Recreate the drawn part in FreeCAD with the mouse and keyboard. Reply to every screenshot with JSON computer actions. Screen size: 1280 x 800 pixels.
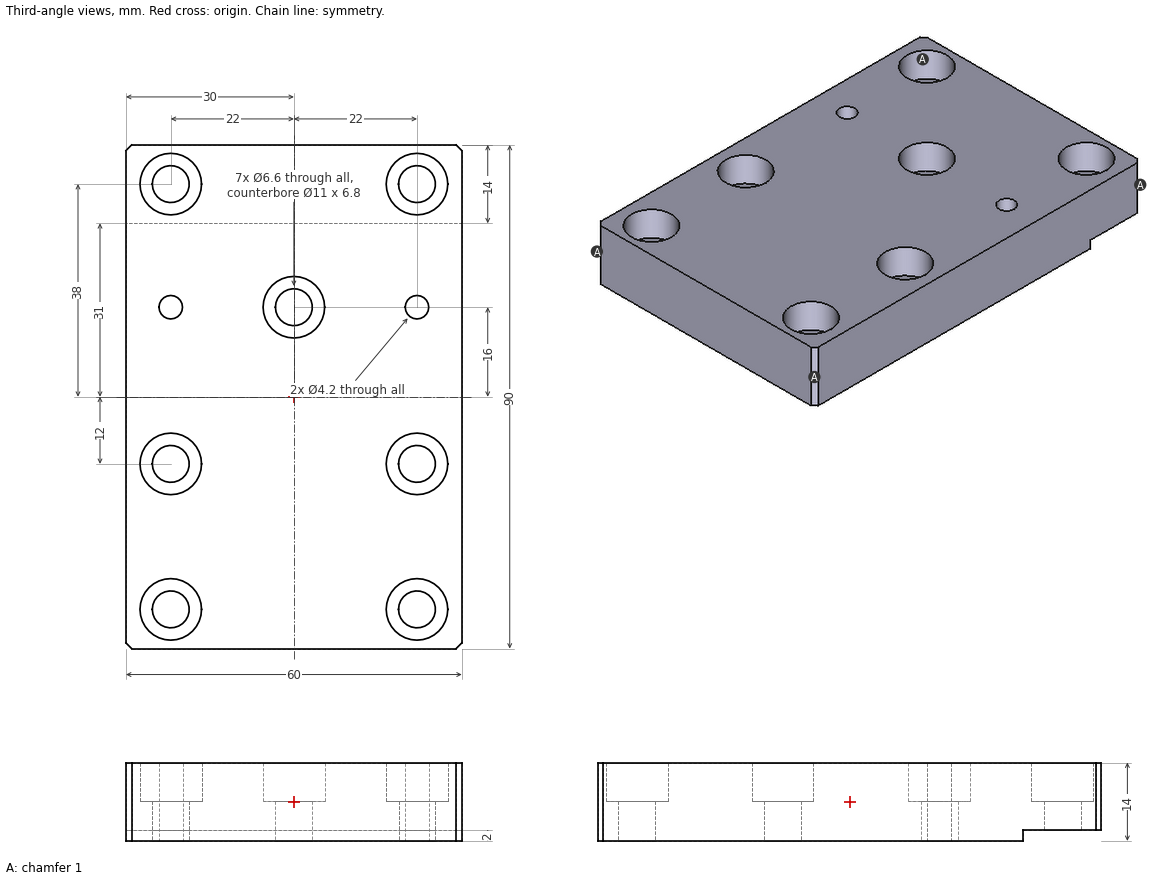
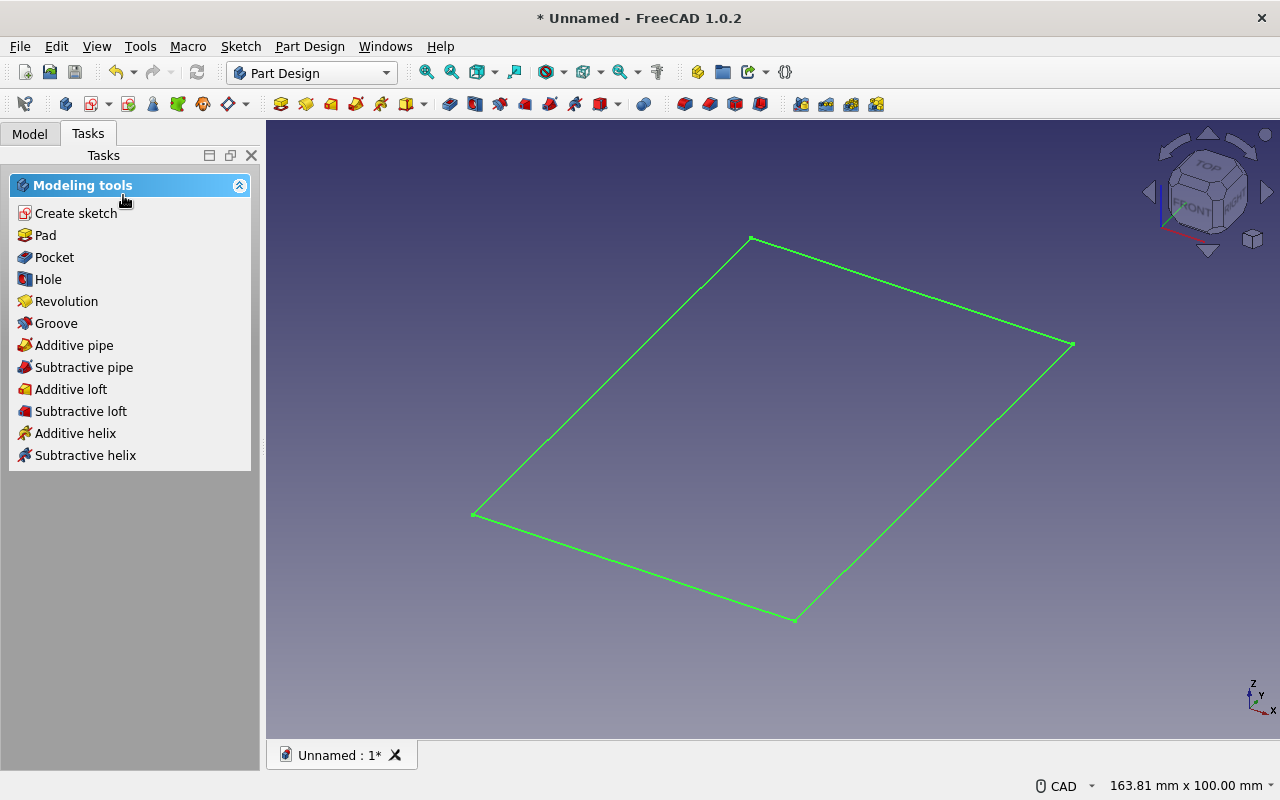
{"action": "left_click", "coordinate": [281, 104]}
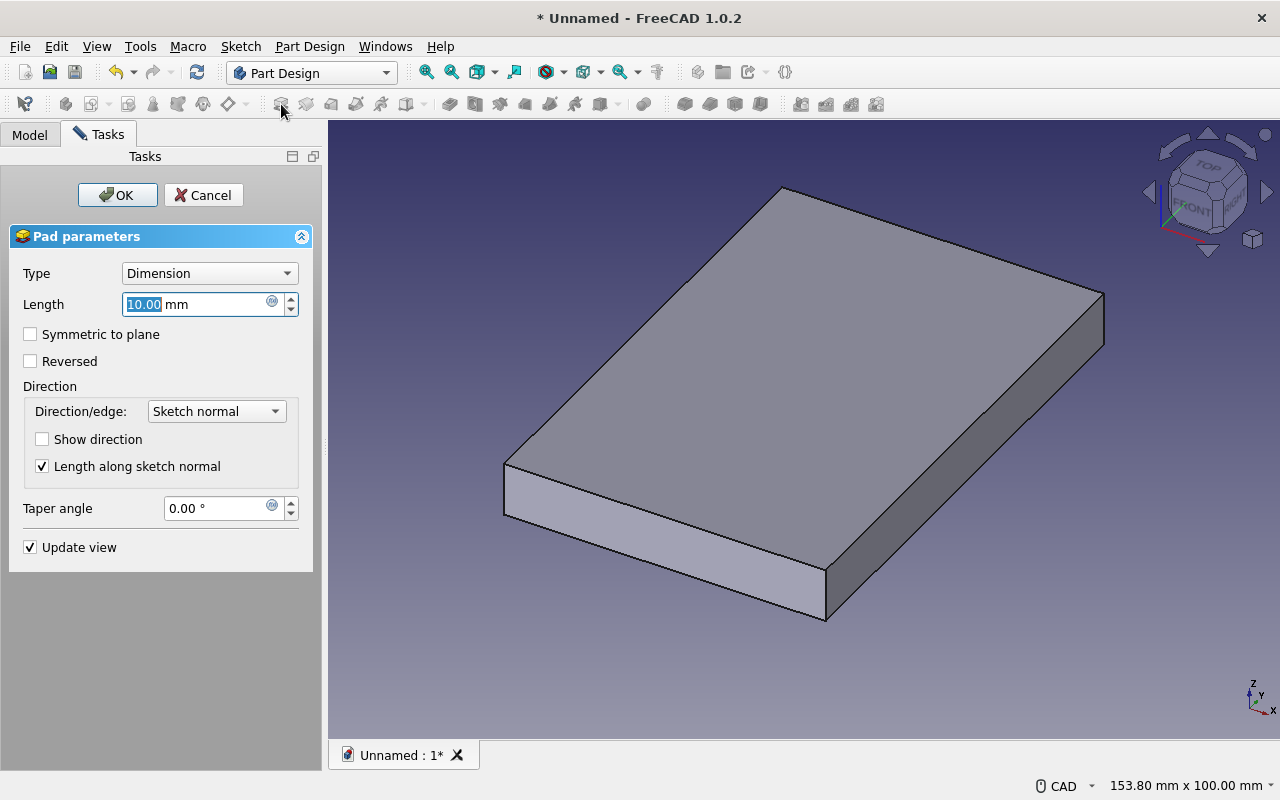
{"action": "type", "text": "14"}
{"action": "key", "text": "Tab"}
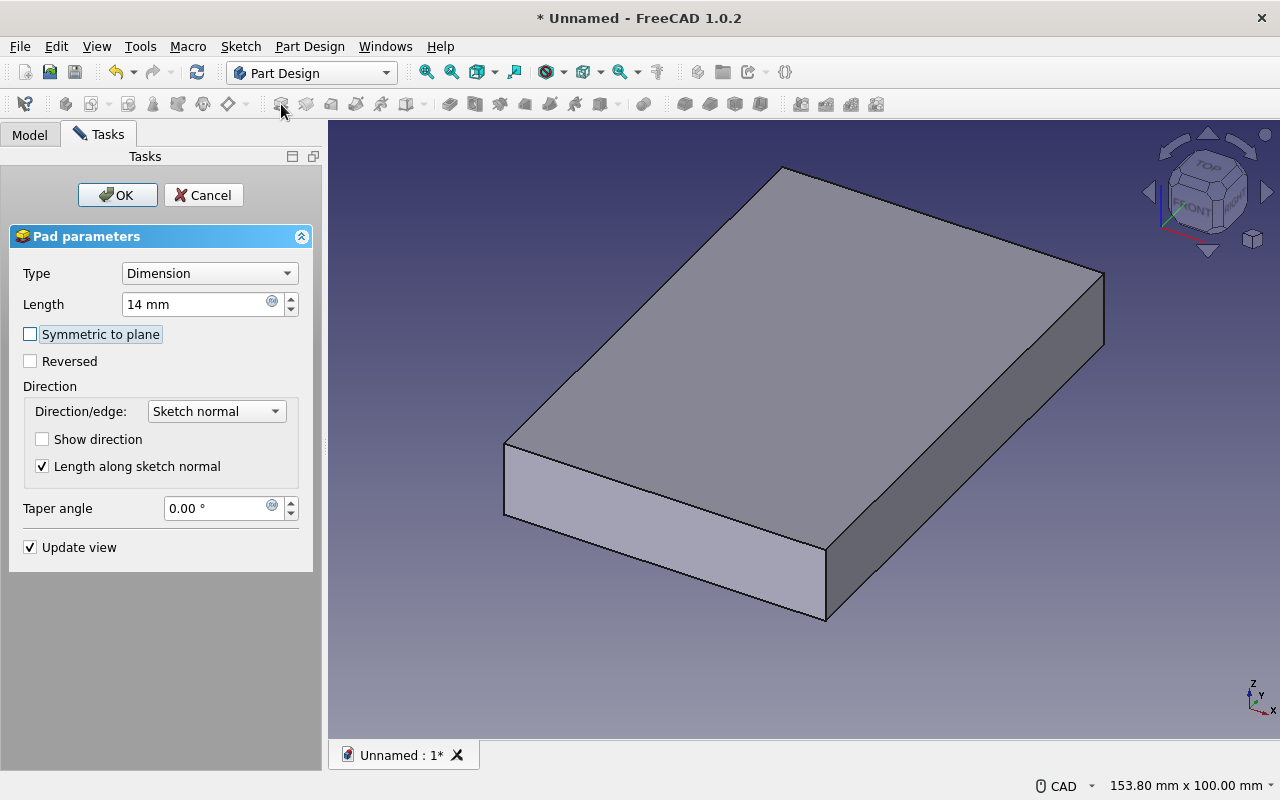
{"action": "left_click", "coordinate": [31, 334]}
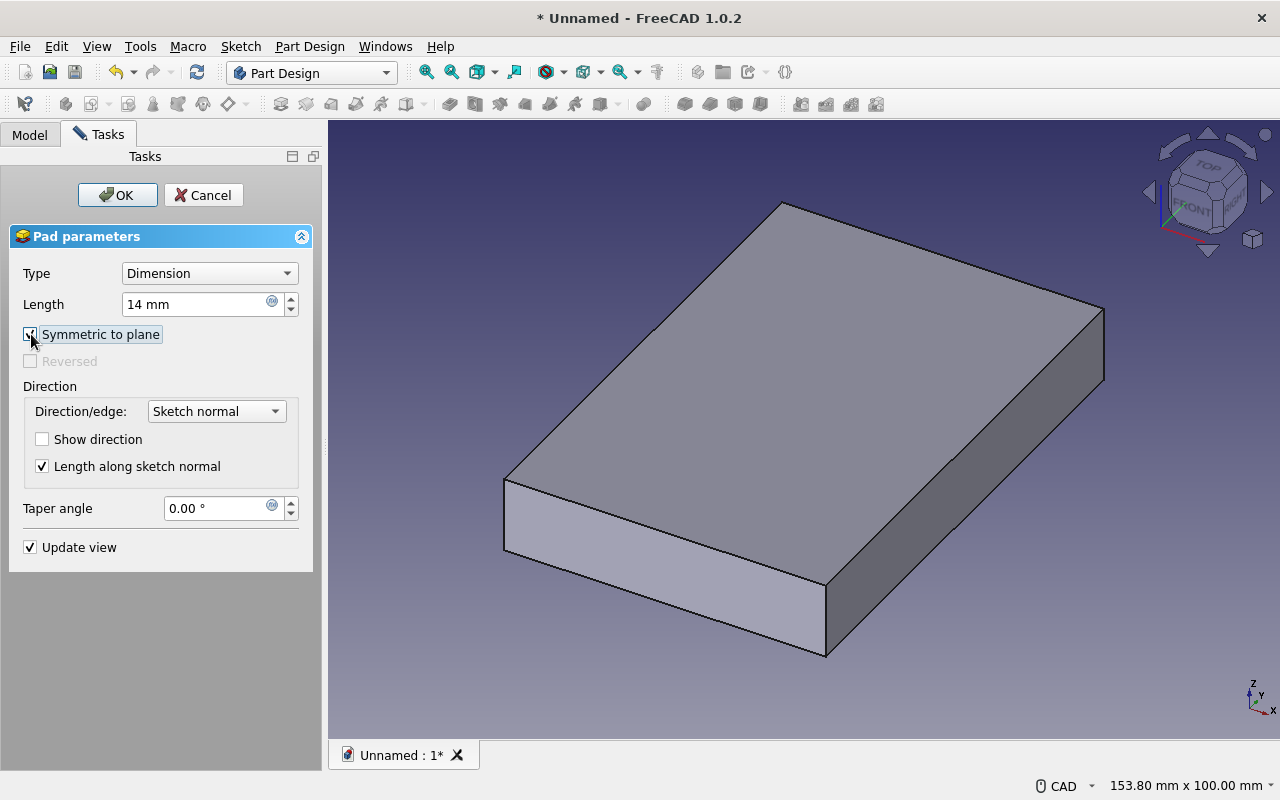
{"action": "left_click", "coordinate": [118, 195]}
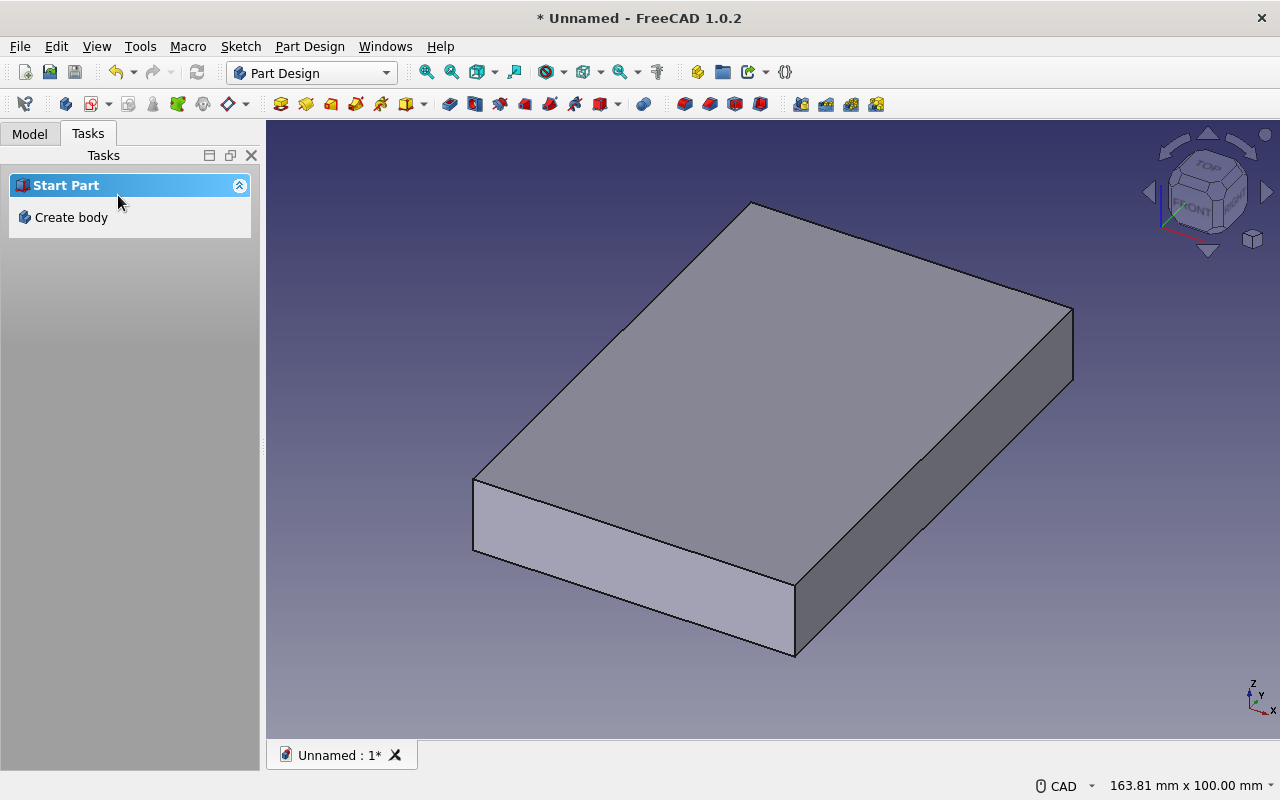
{"action": "key", "text": "5"}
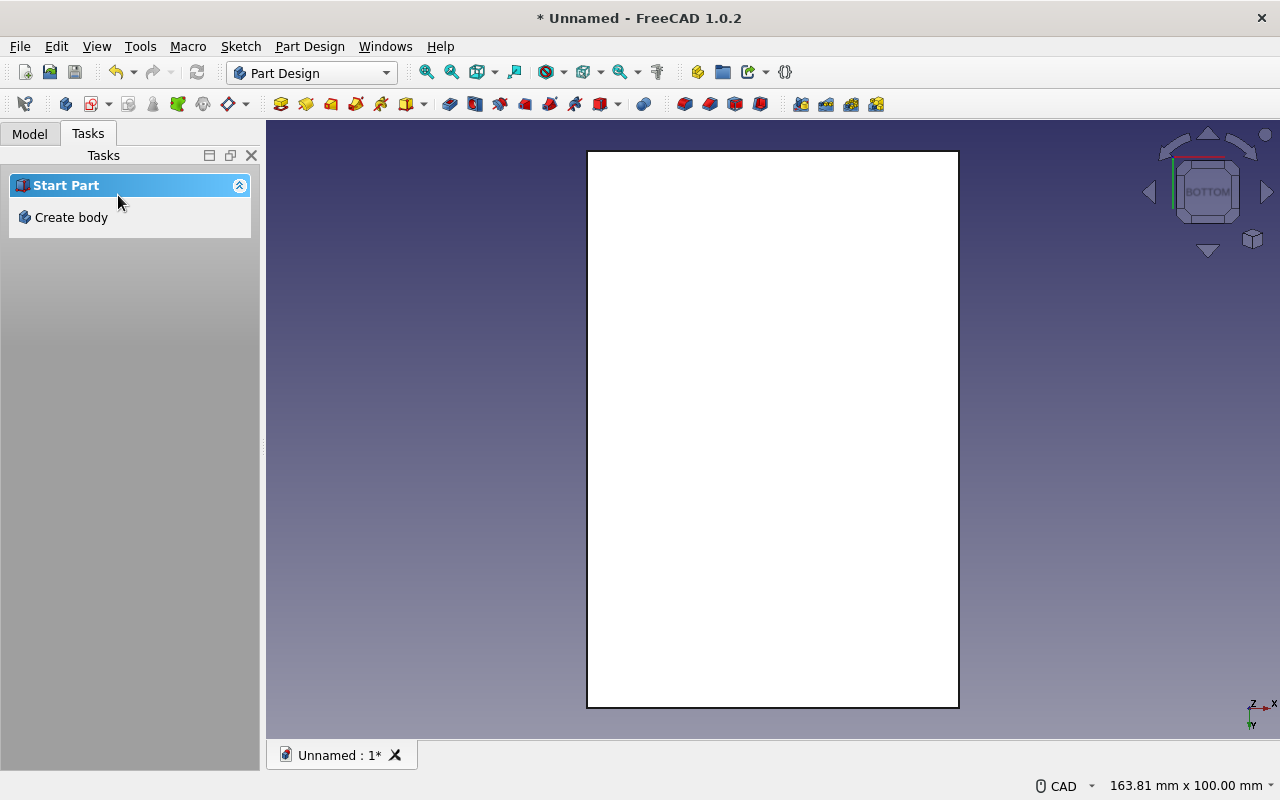
{"action": "left_click", "coordinate": [773, 508]}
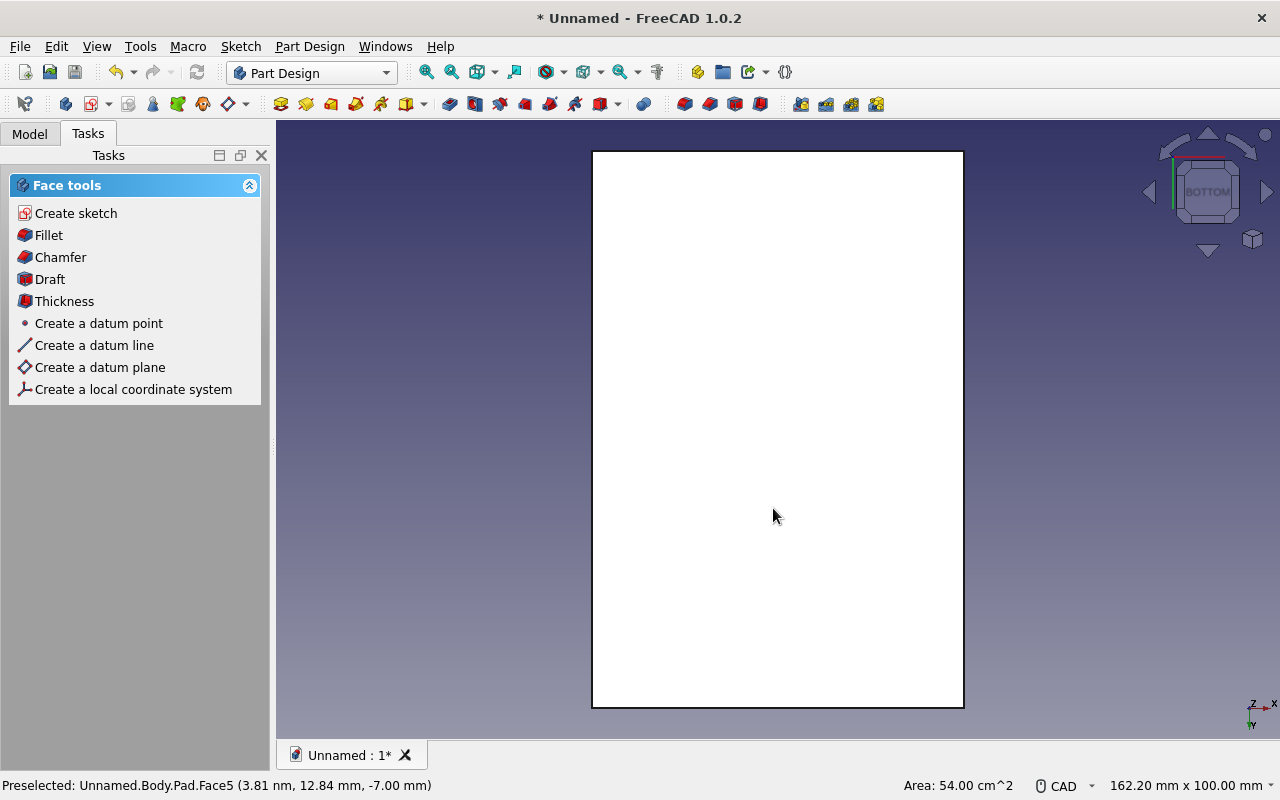
{"action": "left_click", "coordinate": [90, 104]}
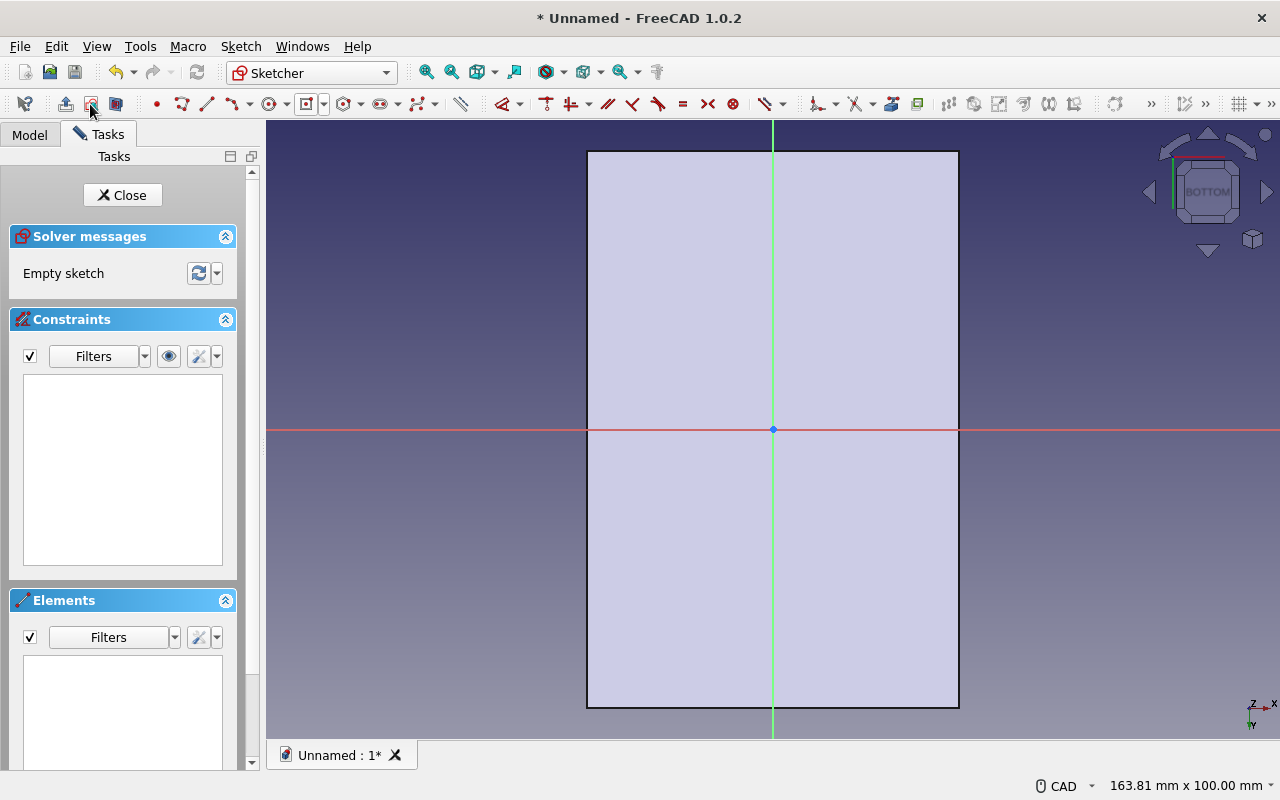
{"action": "scroll", "coordinate": [395, 148], "scroll_direction": "down", "scroll_amount": 1}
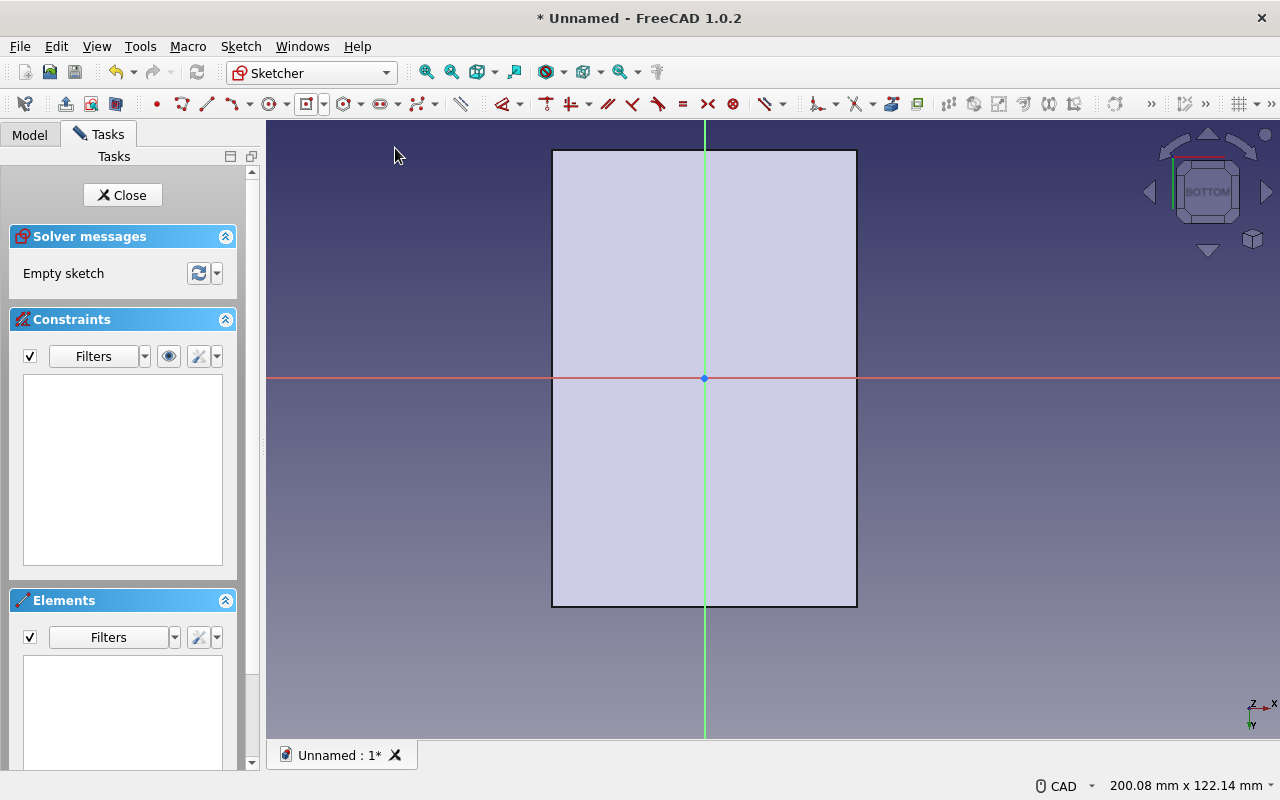
{"action": "scroll", "coordinate": [705, 569], "scroll_direction": "up", "scroll_amount": 3}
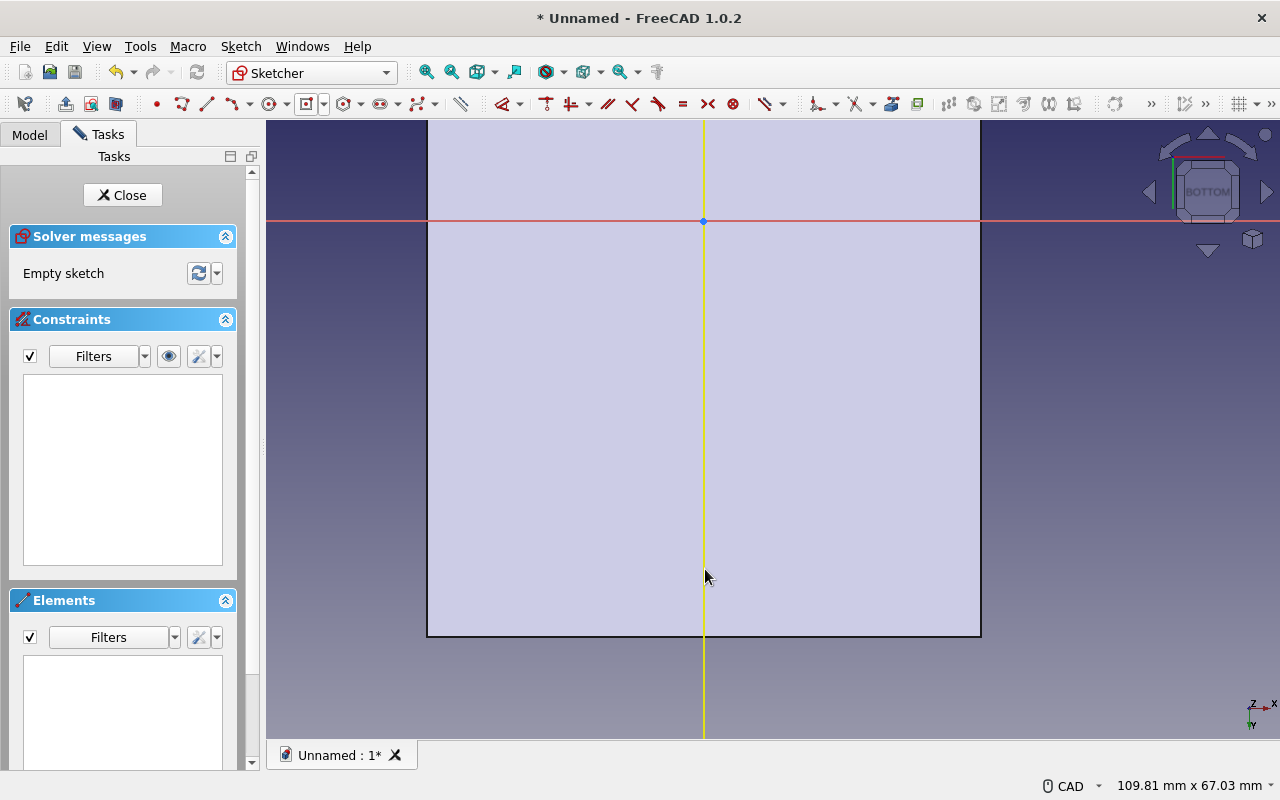
{"action": "left_click", "coordinate": [324, 104]}